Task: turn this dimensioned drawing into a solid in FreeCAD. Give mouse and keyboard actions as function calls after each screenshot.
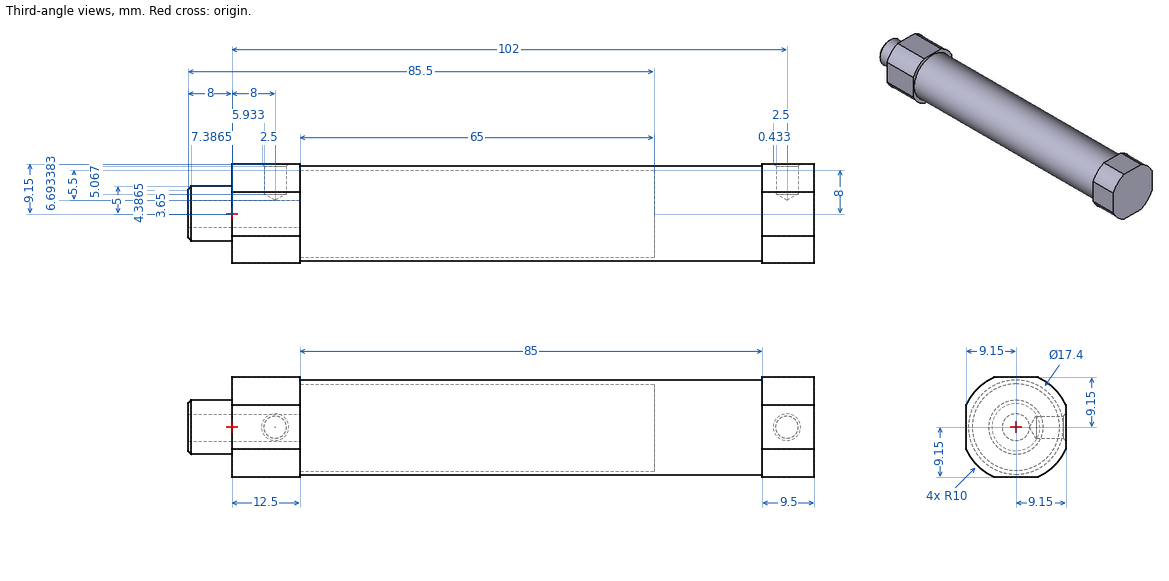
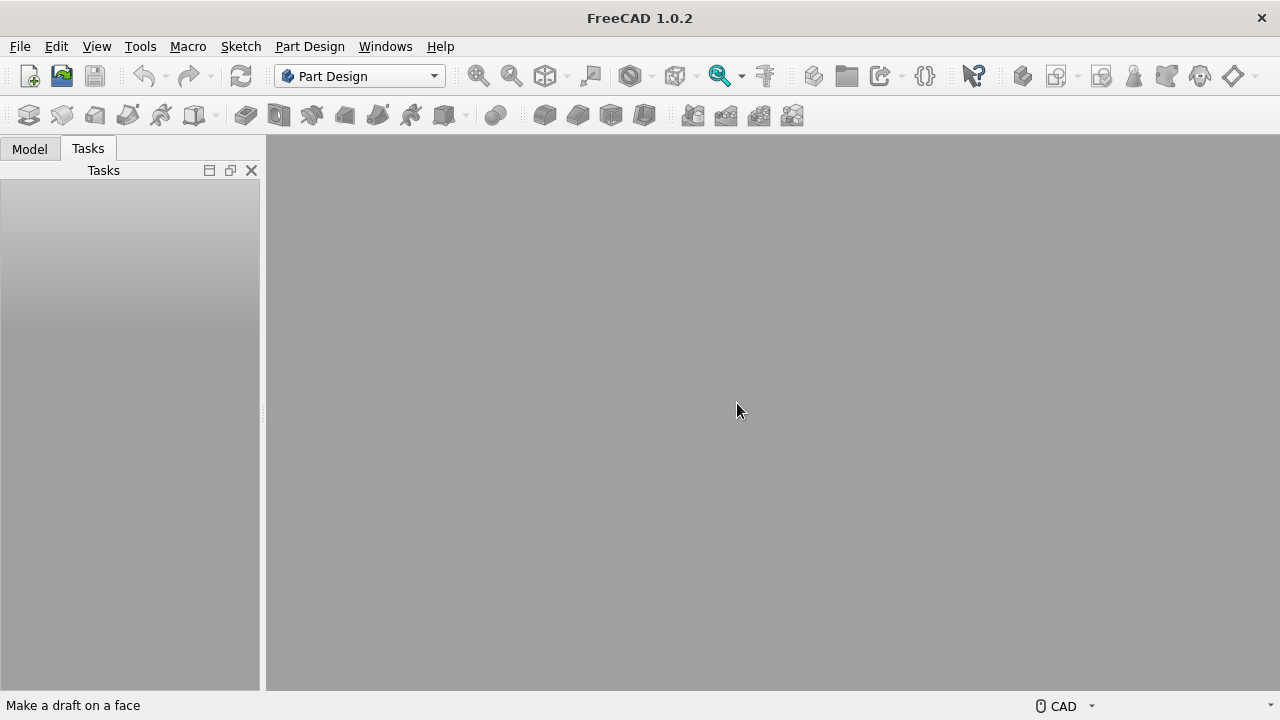
click(29, 76)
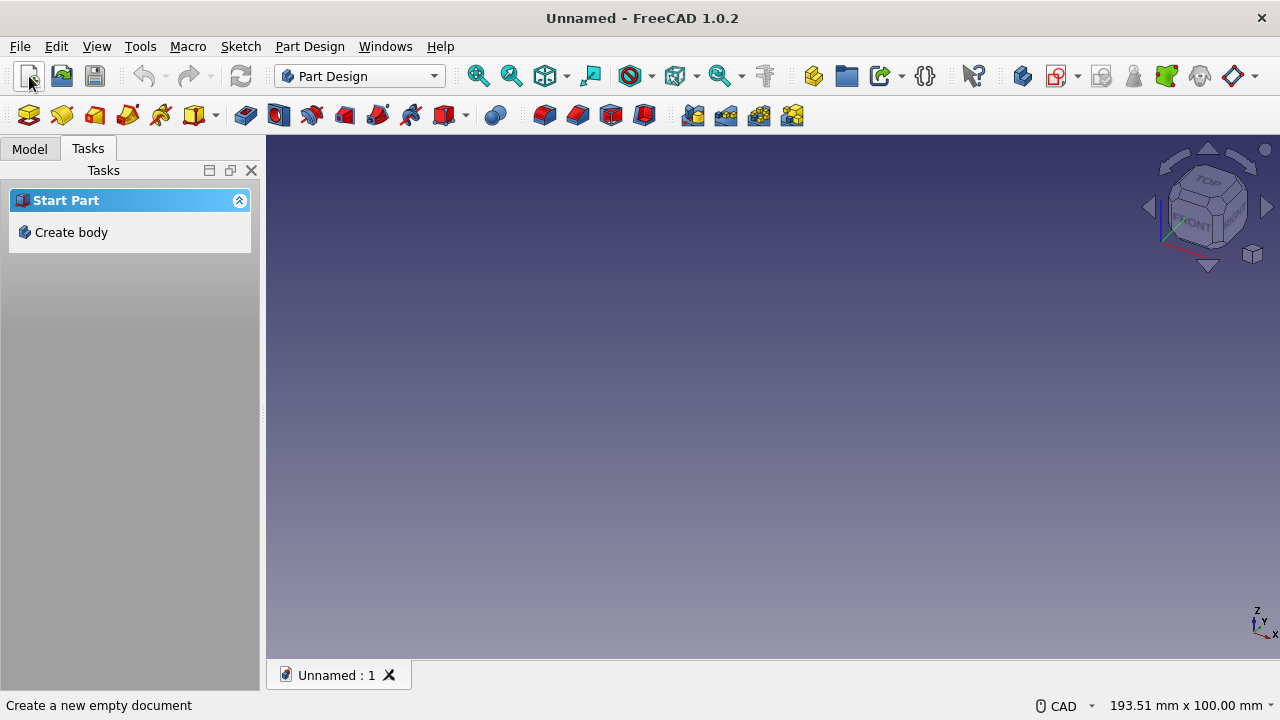
click(1056, 76)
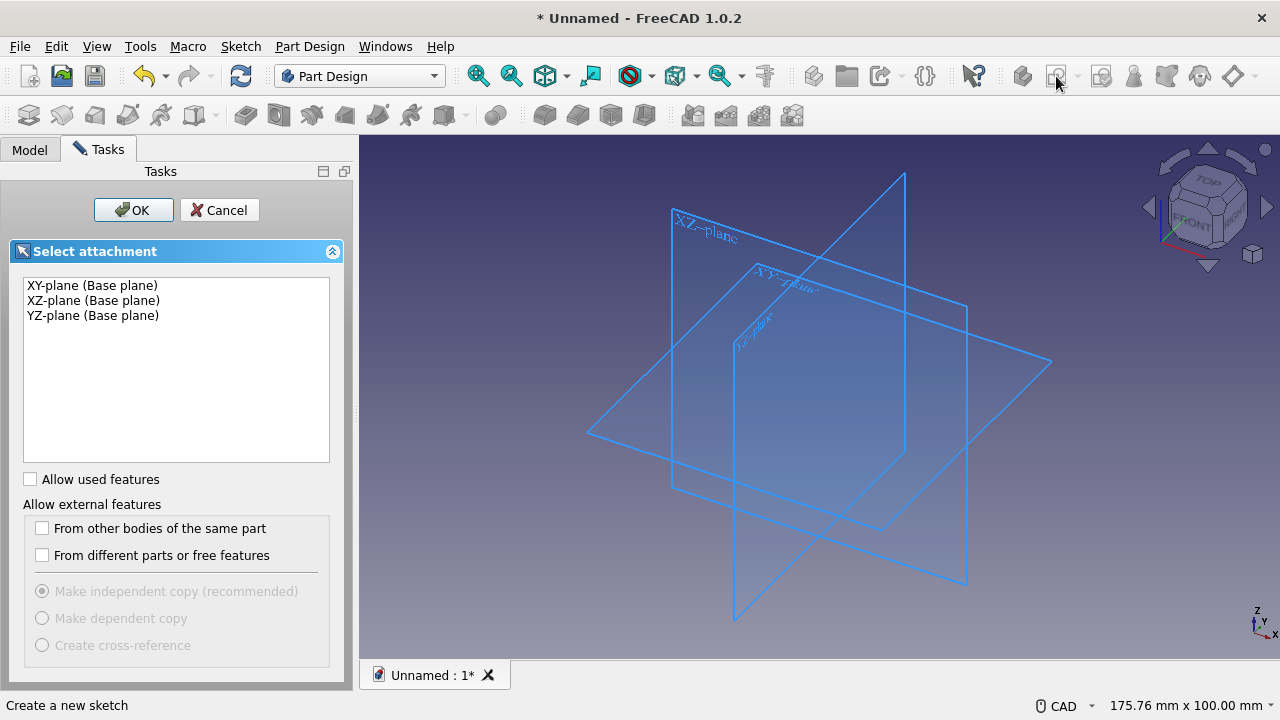
click(84, 286)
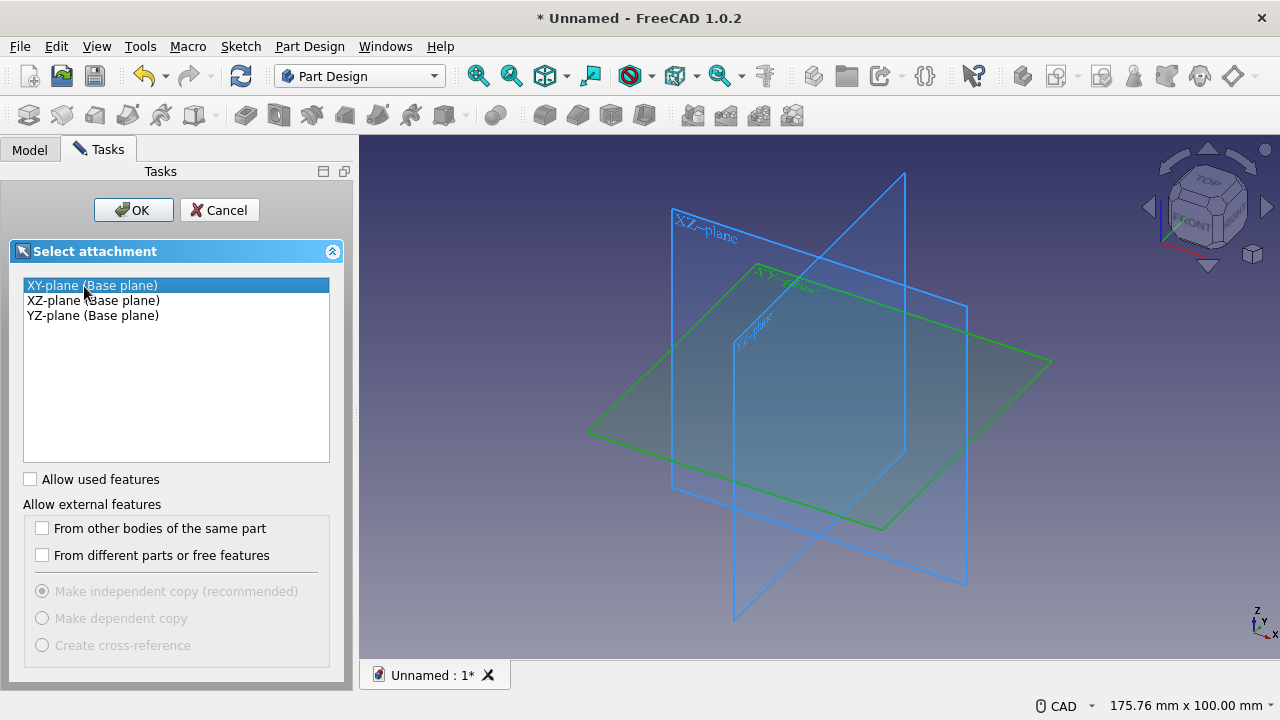
click(134, 210)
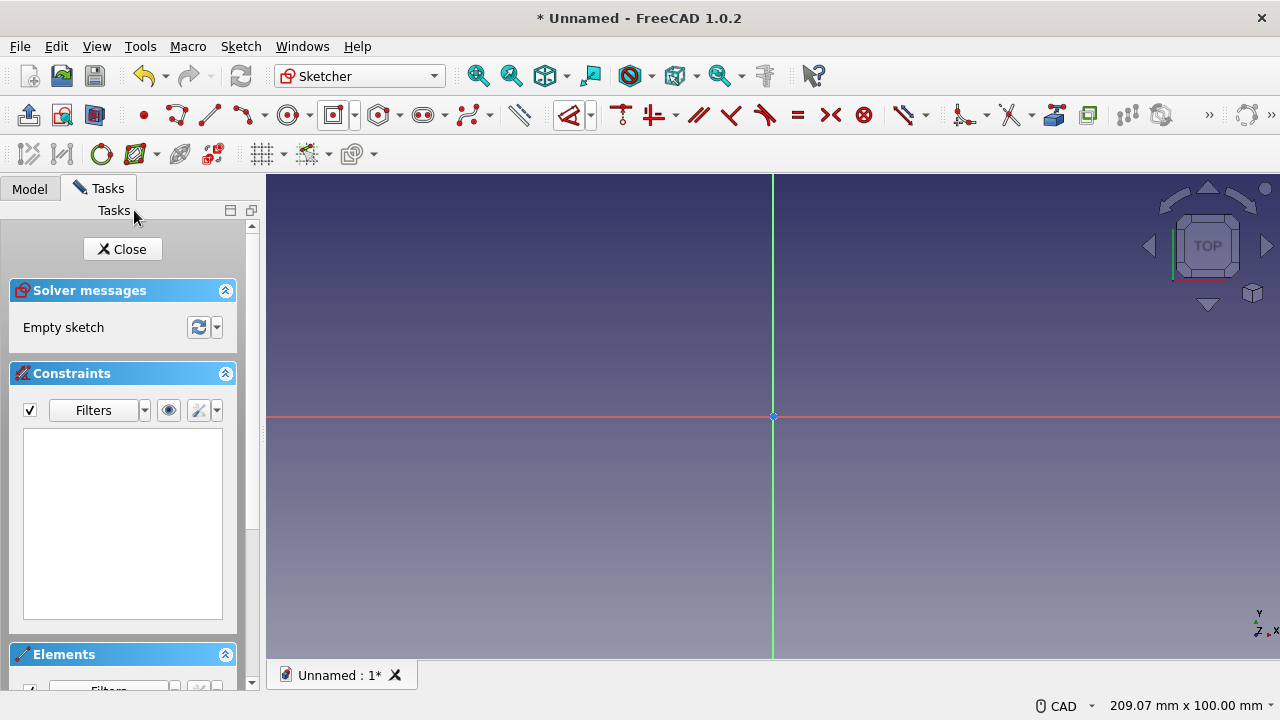
scroll(758, 403, up, 13)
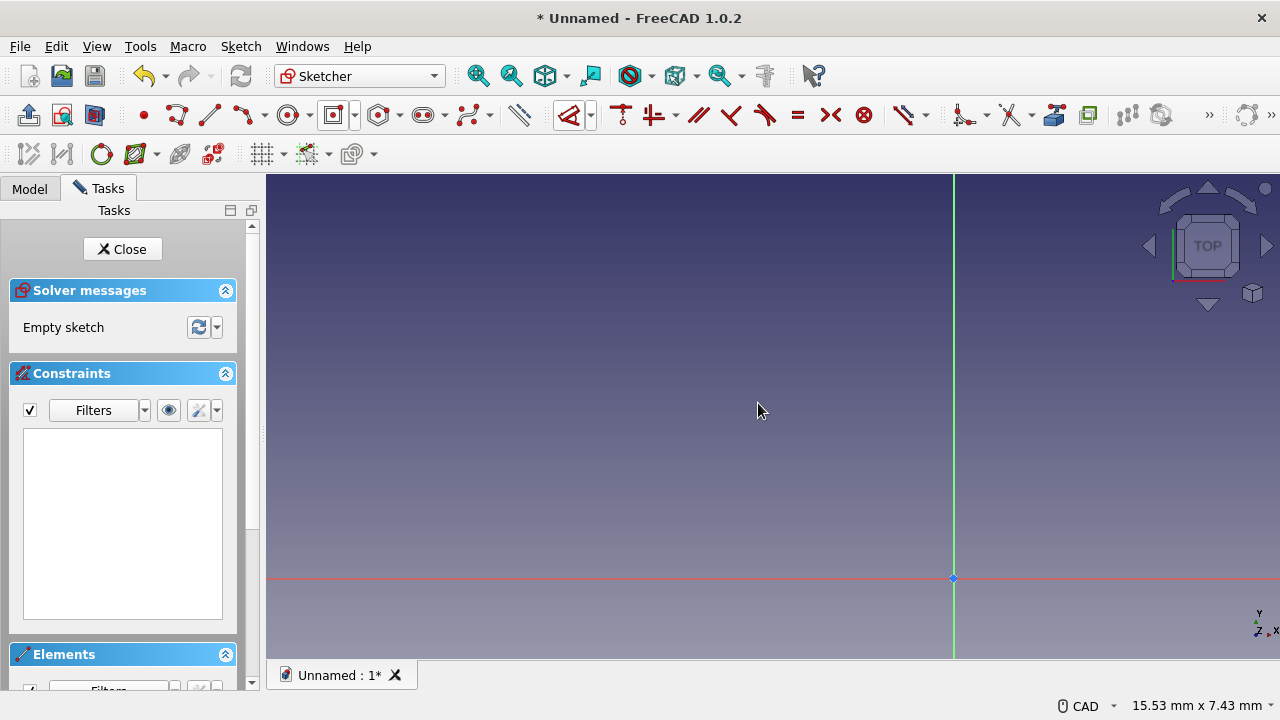
click(177, 116)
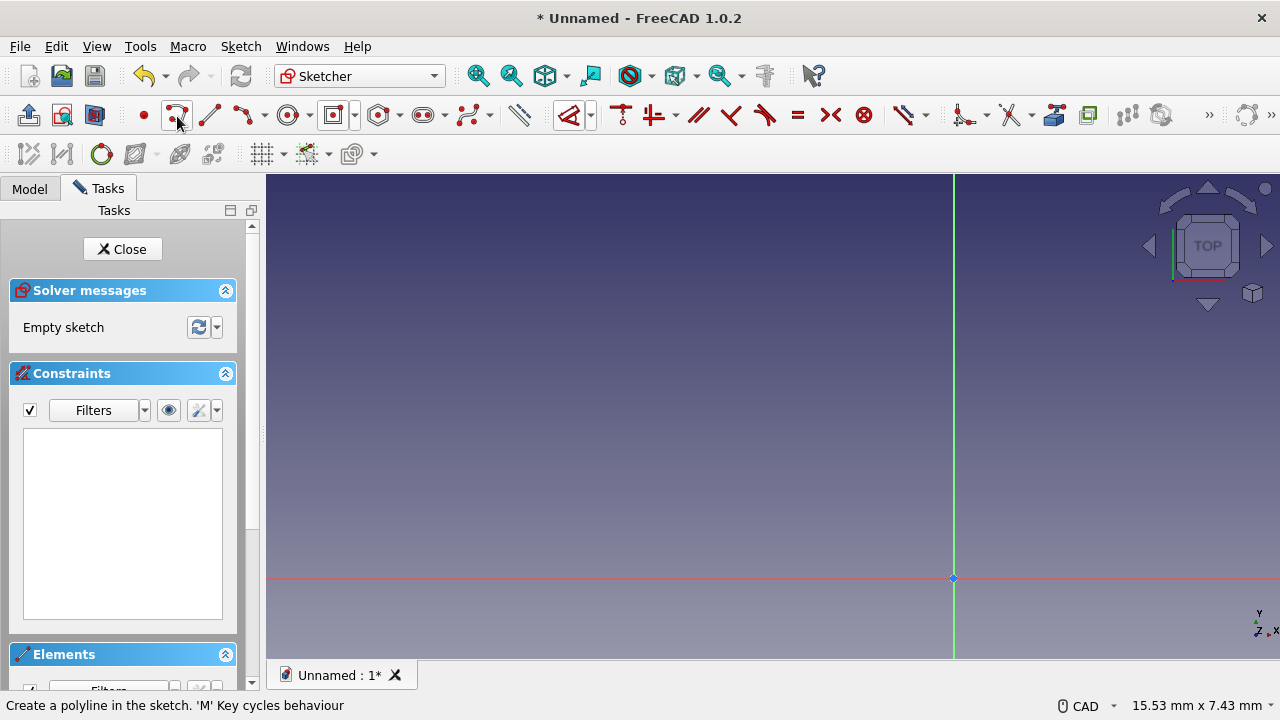
click(954, 579)
click(945, 252)
click(472, 252)
click(432, 292)
click(432, 570)
click(954, 579)
key(Escape)
key(Escape)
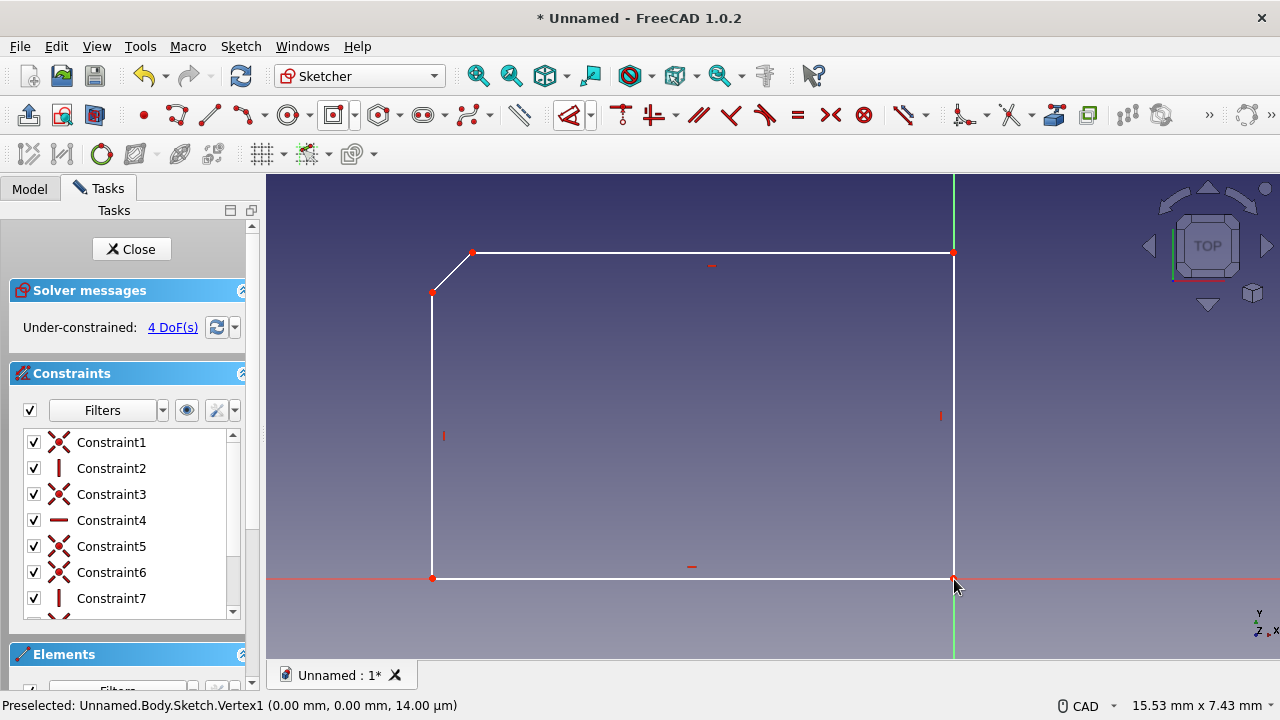
click(568, 116)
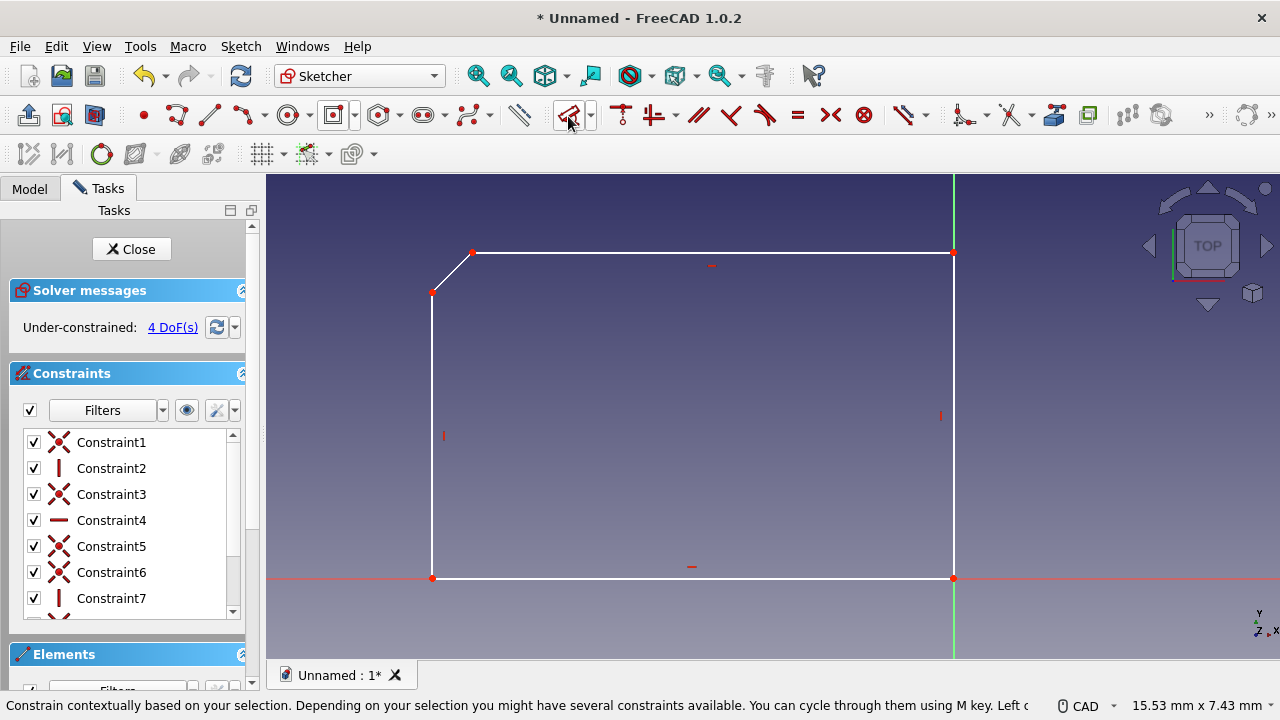
click(954, 481)
click(988, 416)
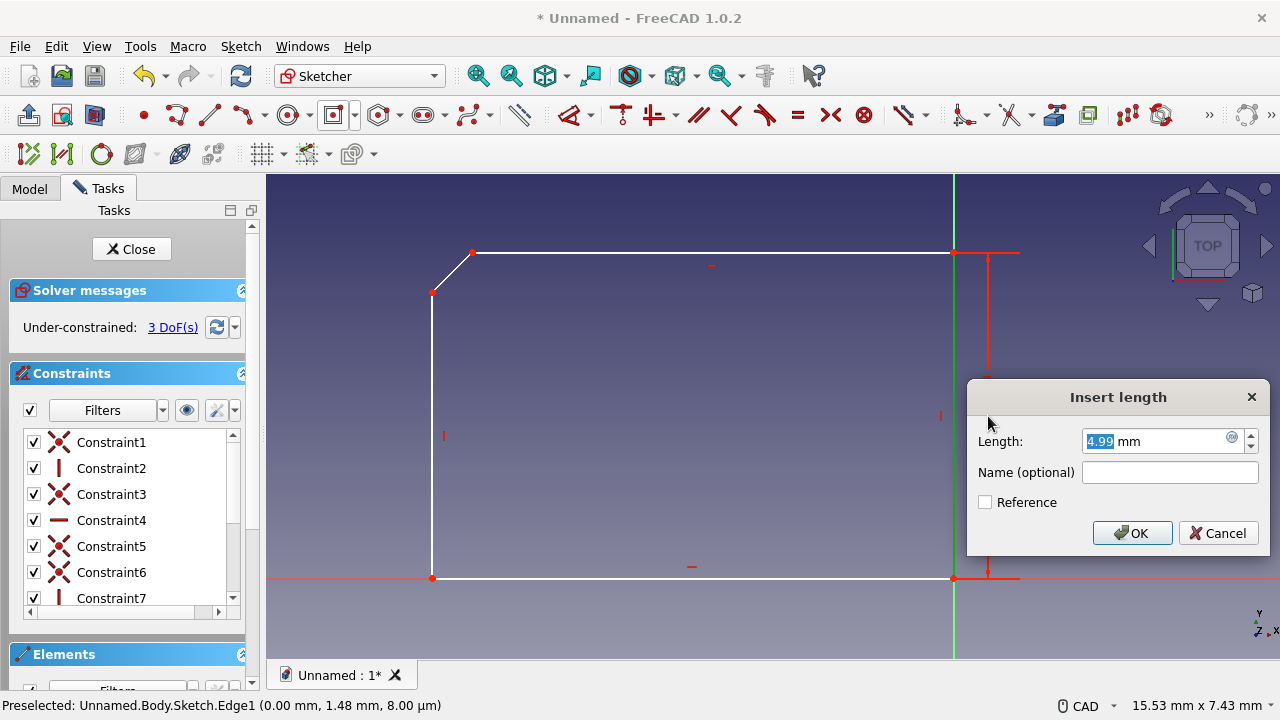
text(5)
key(Return)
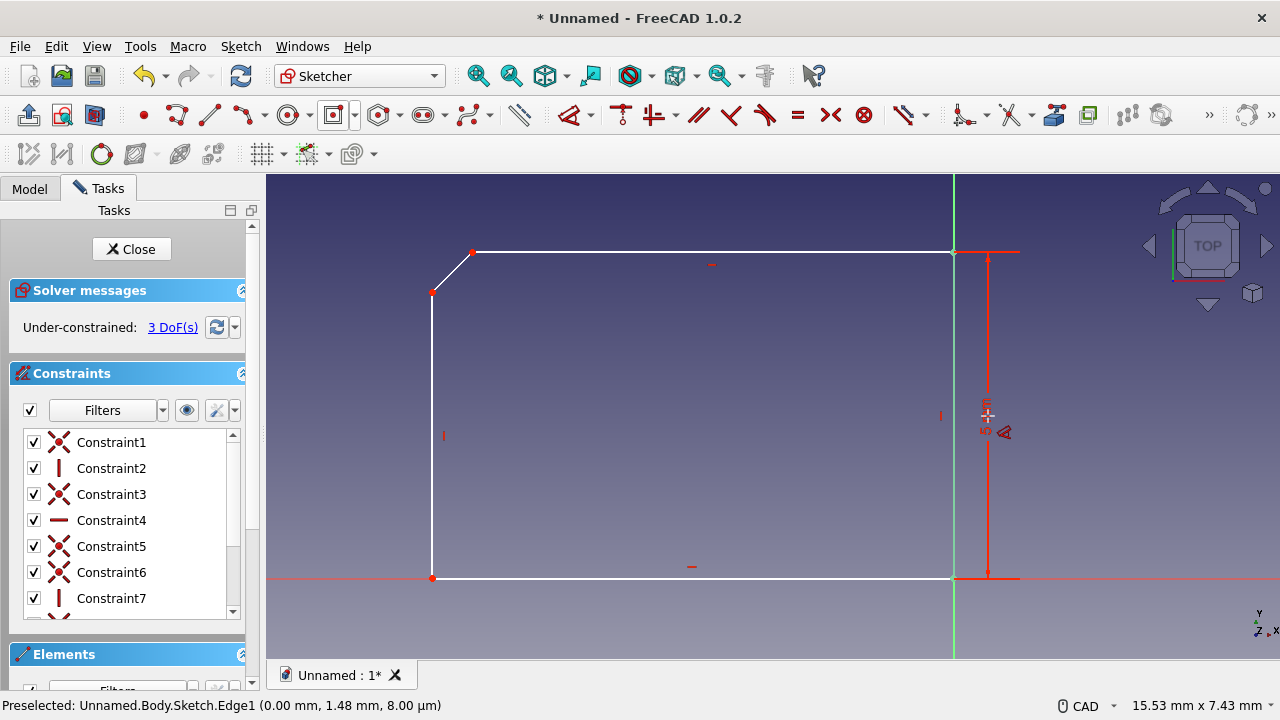
click(589, 579)
click(693, 613)